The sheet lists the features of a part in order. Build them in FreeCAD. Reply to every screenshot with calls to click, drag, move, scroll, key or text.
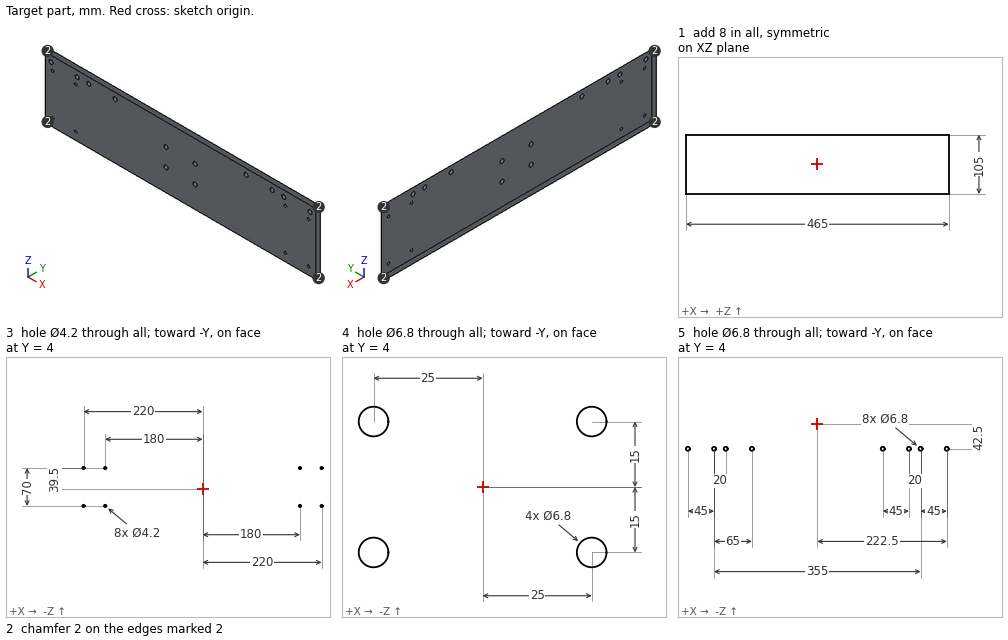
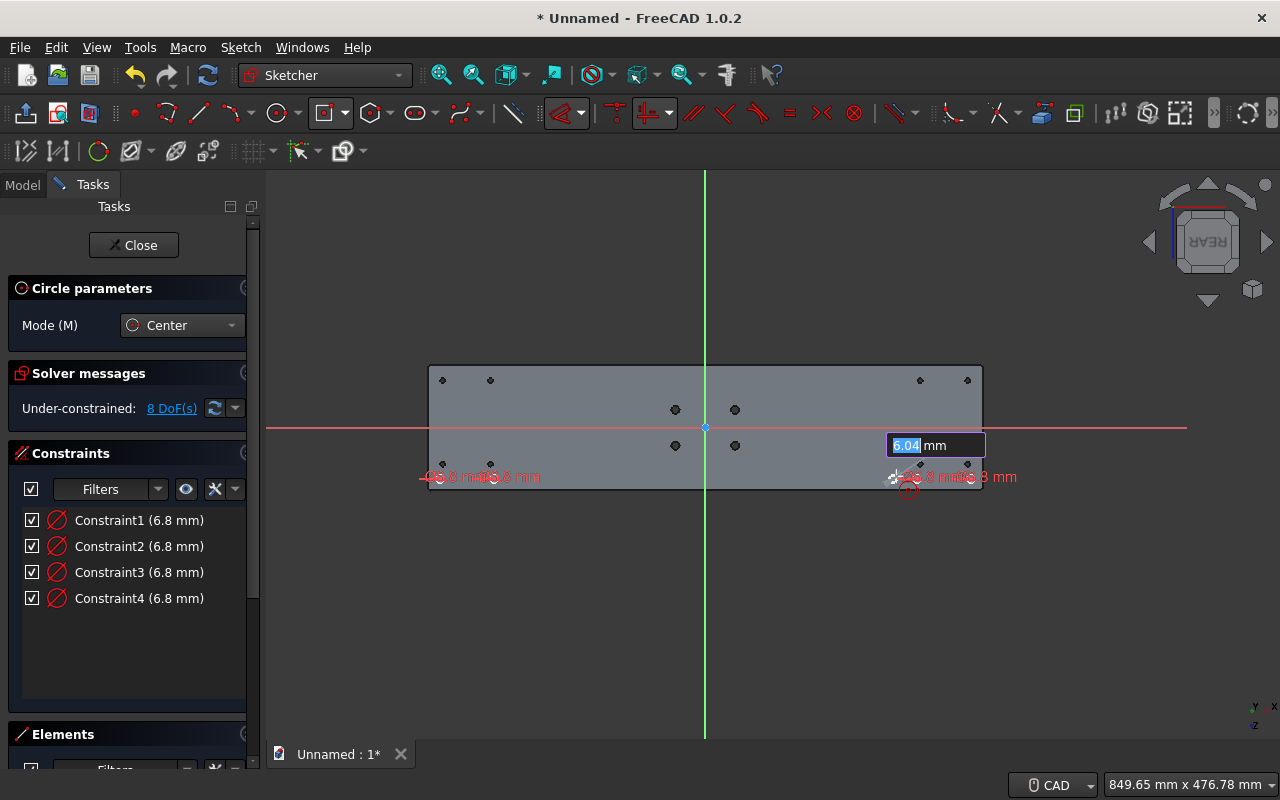
text(6.8)
key(Return)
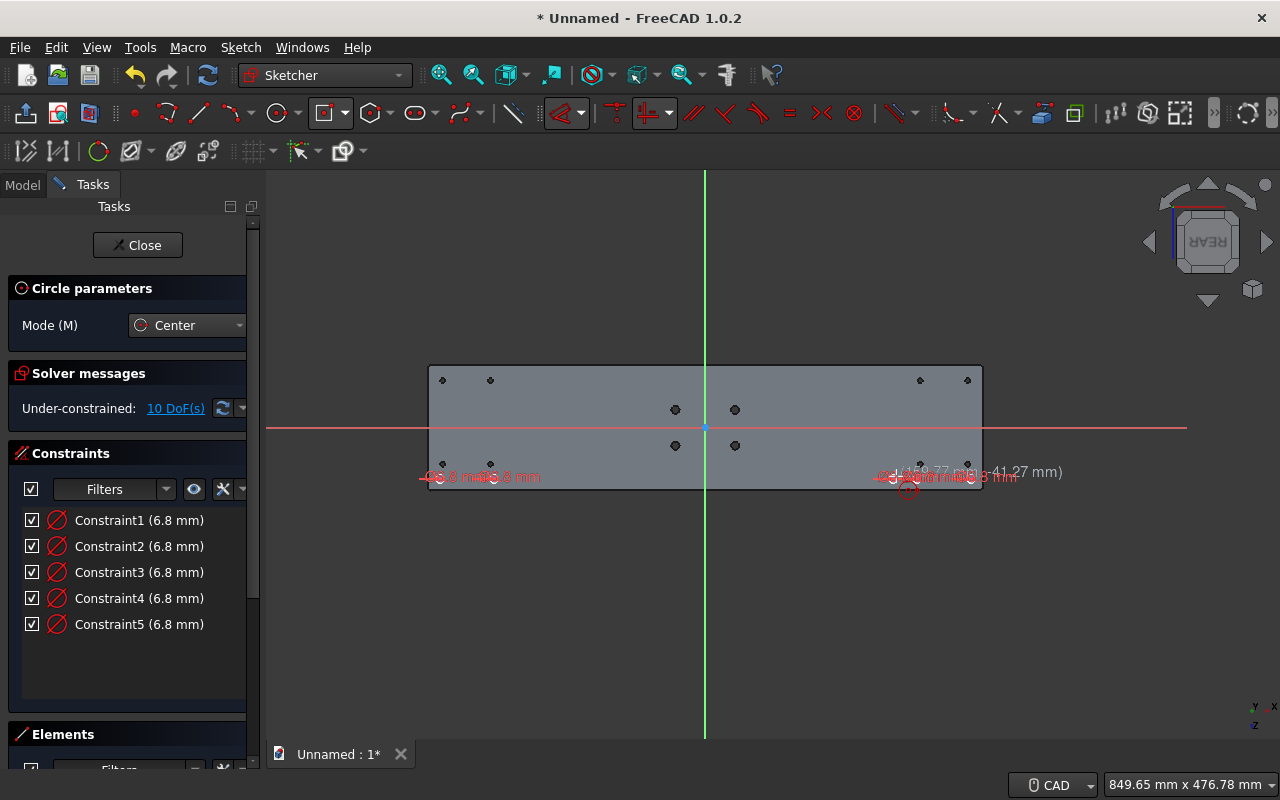
scroll(840, 478, up, 9)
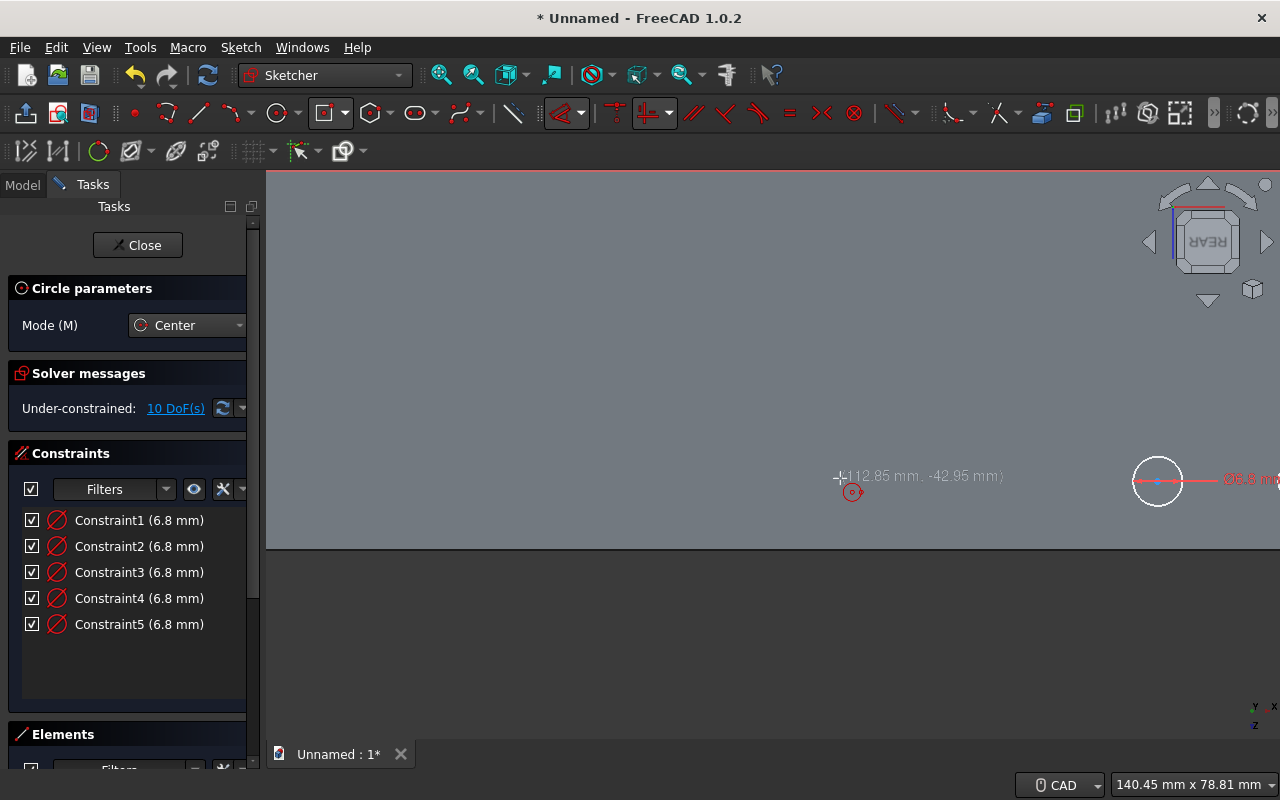
scroll(840, 478, down, 9)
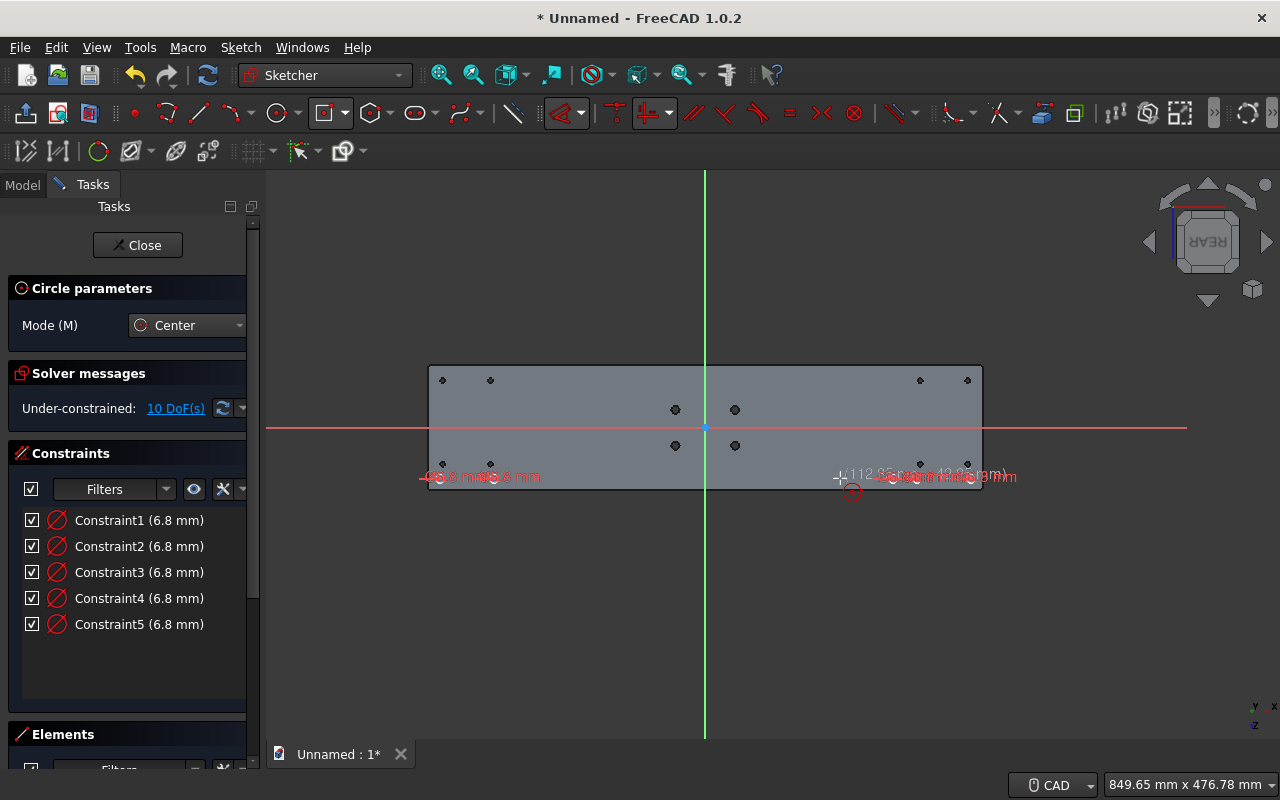
click(840, 478)
move(842, 476)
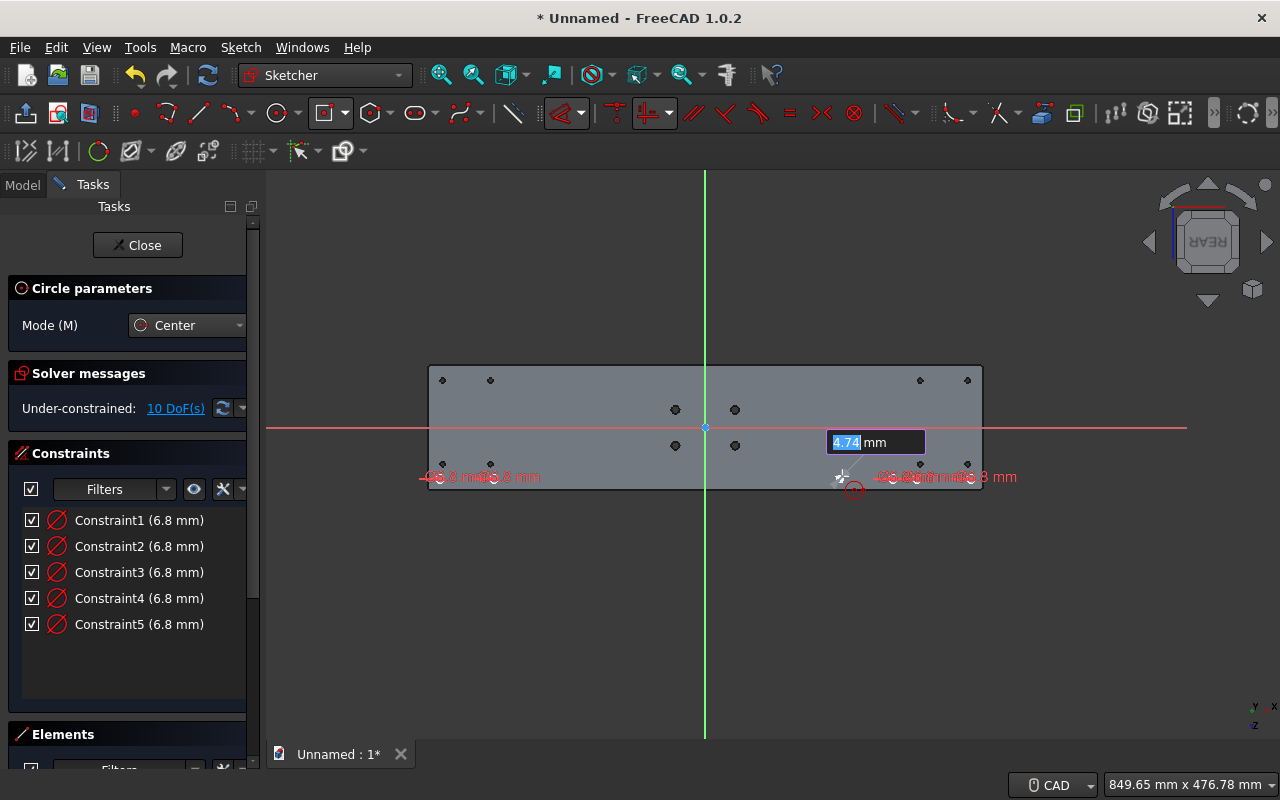
text(6.8)
key(Return)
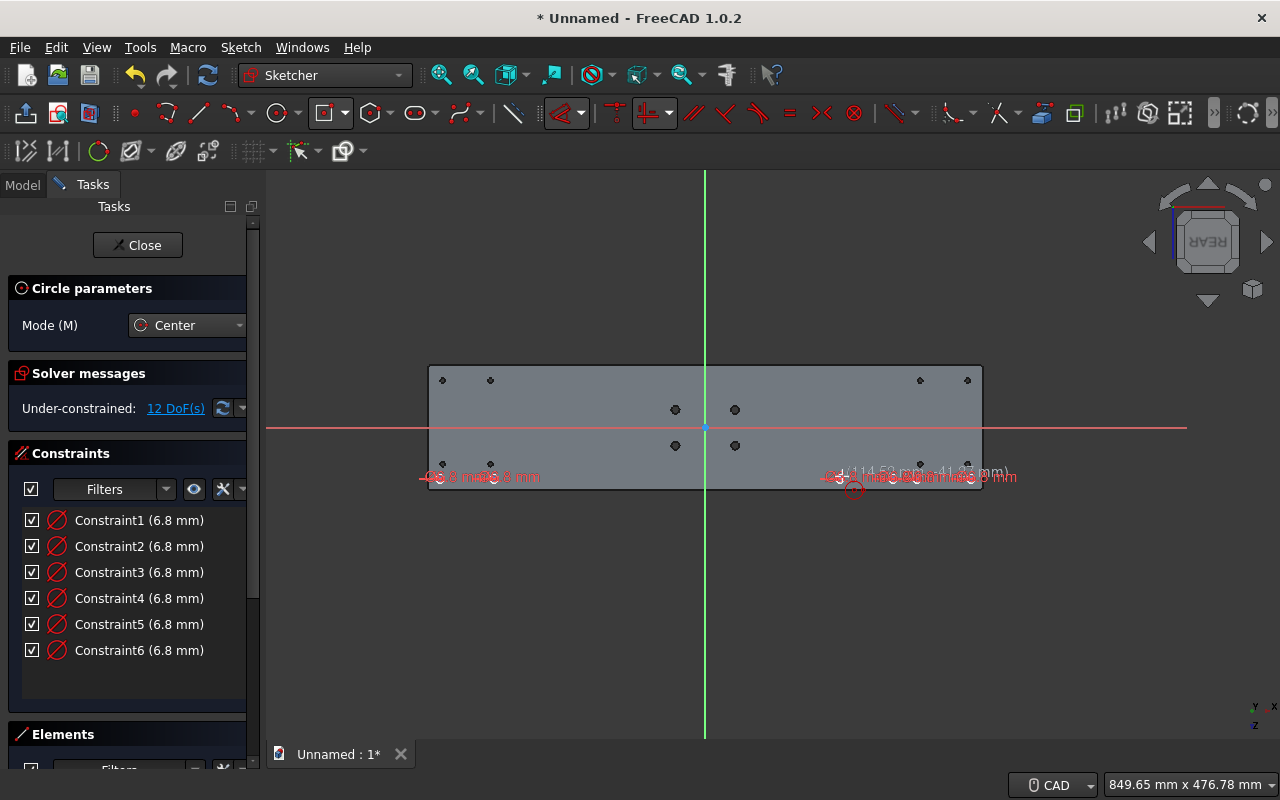
scroll(571, 478, up, 9)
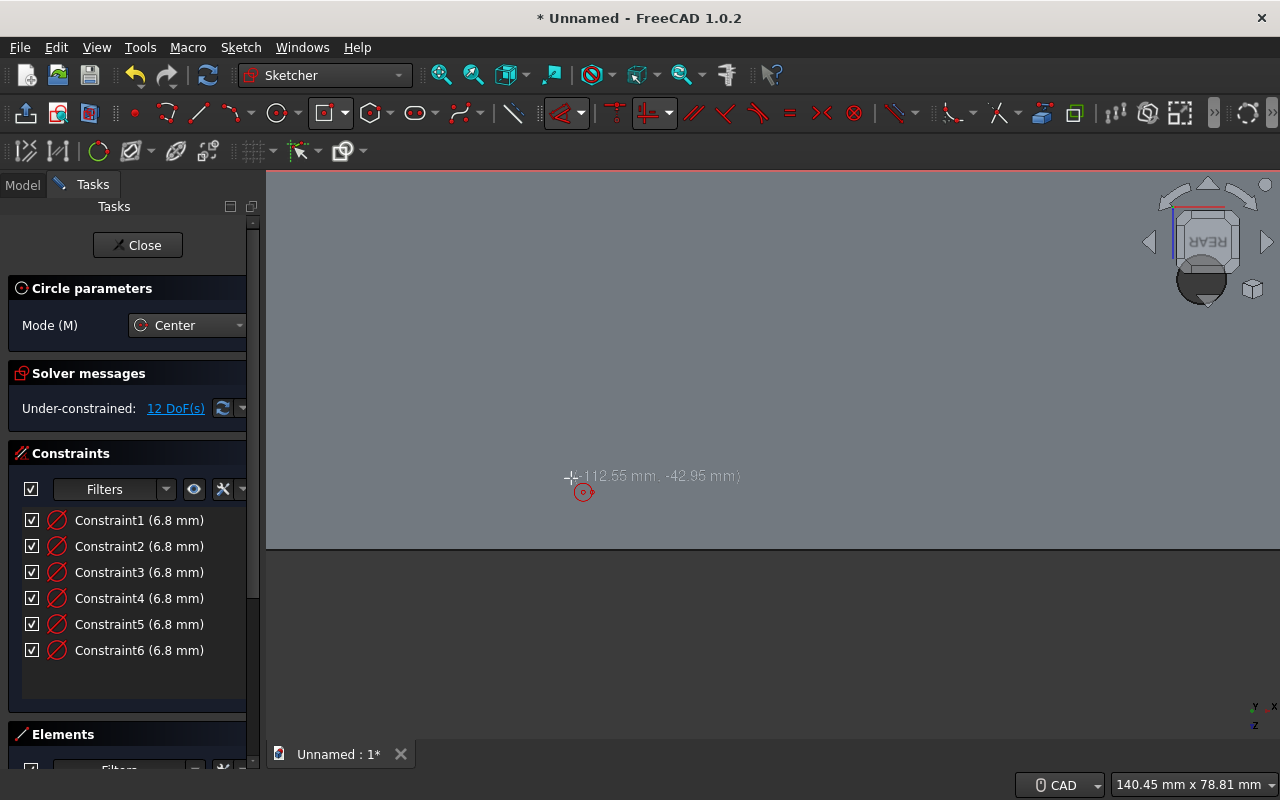
scroll(570, 478, down, 9)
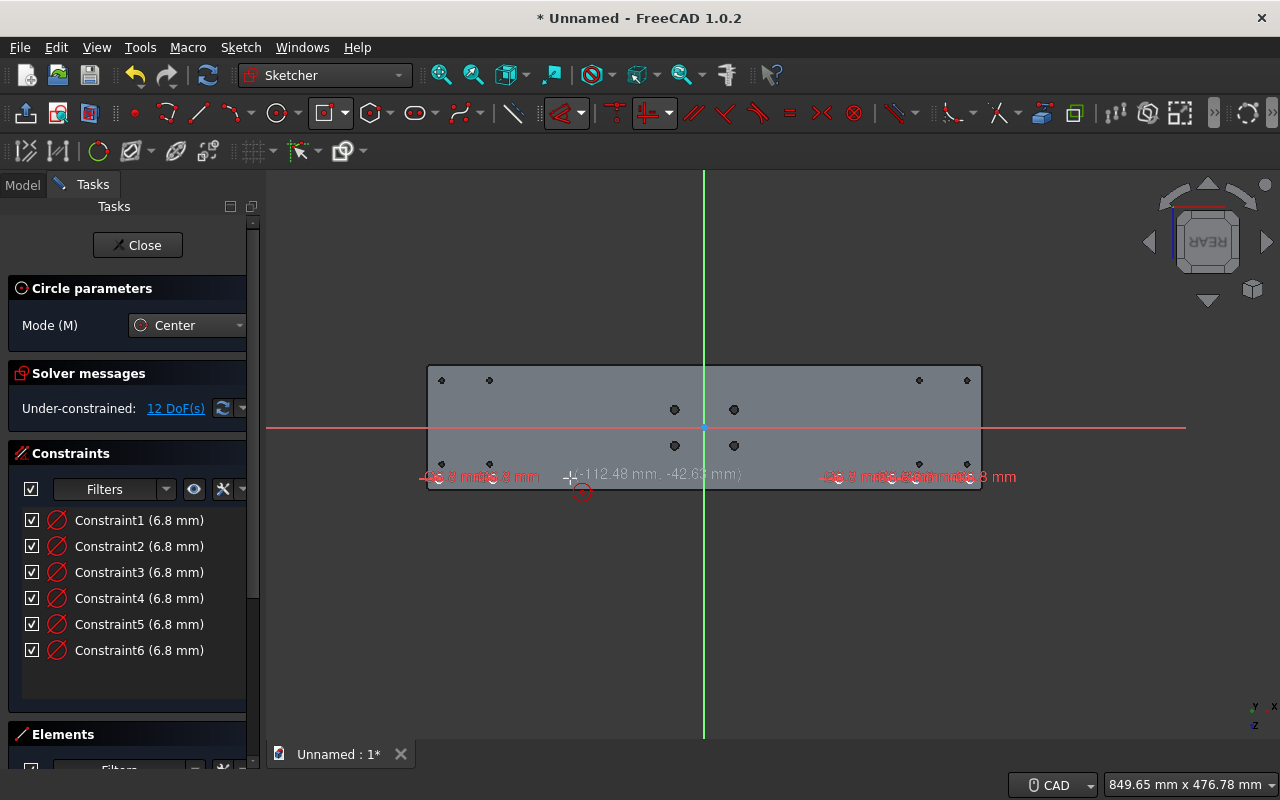
click(570, 478)
move(573, 476)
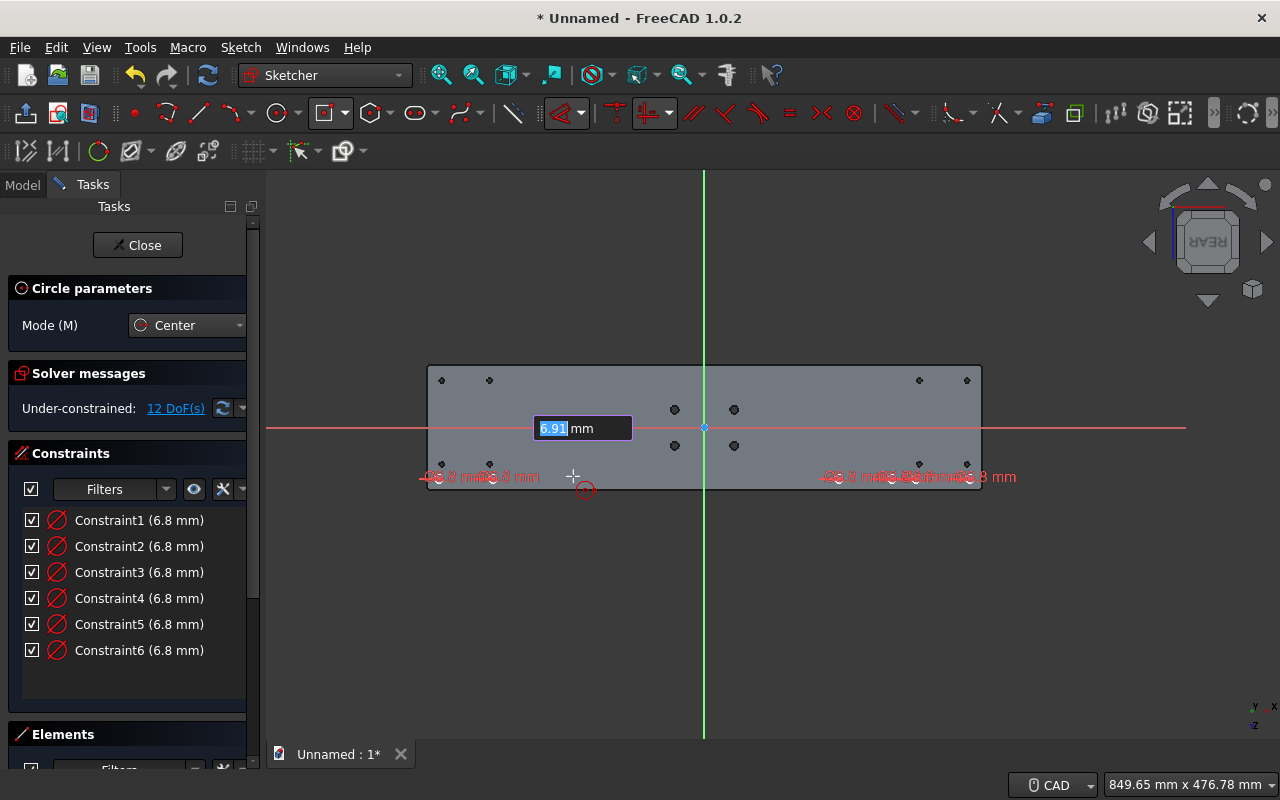
text(6.8)
key(Return)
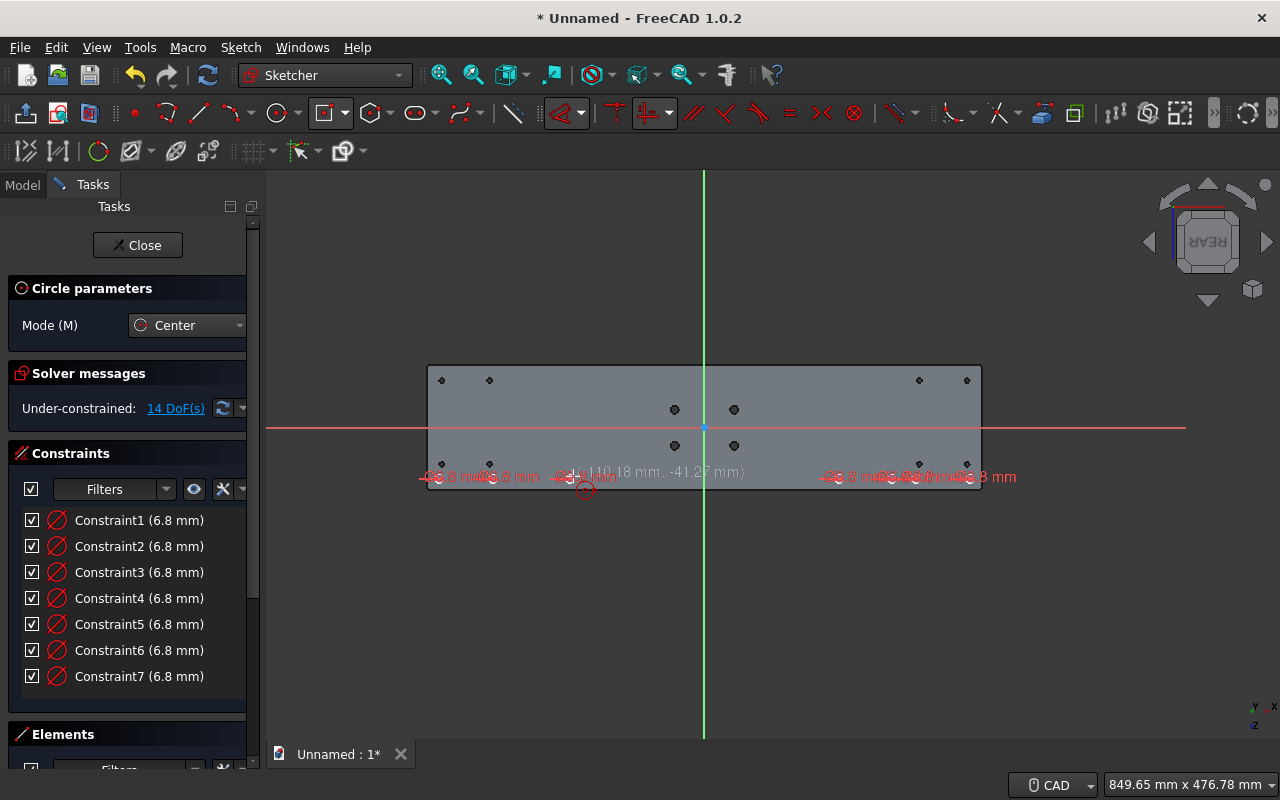
scroll(517, 478, up, 9)